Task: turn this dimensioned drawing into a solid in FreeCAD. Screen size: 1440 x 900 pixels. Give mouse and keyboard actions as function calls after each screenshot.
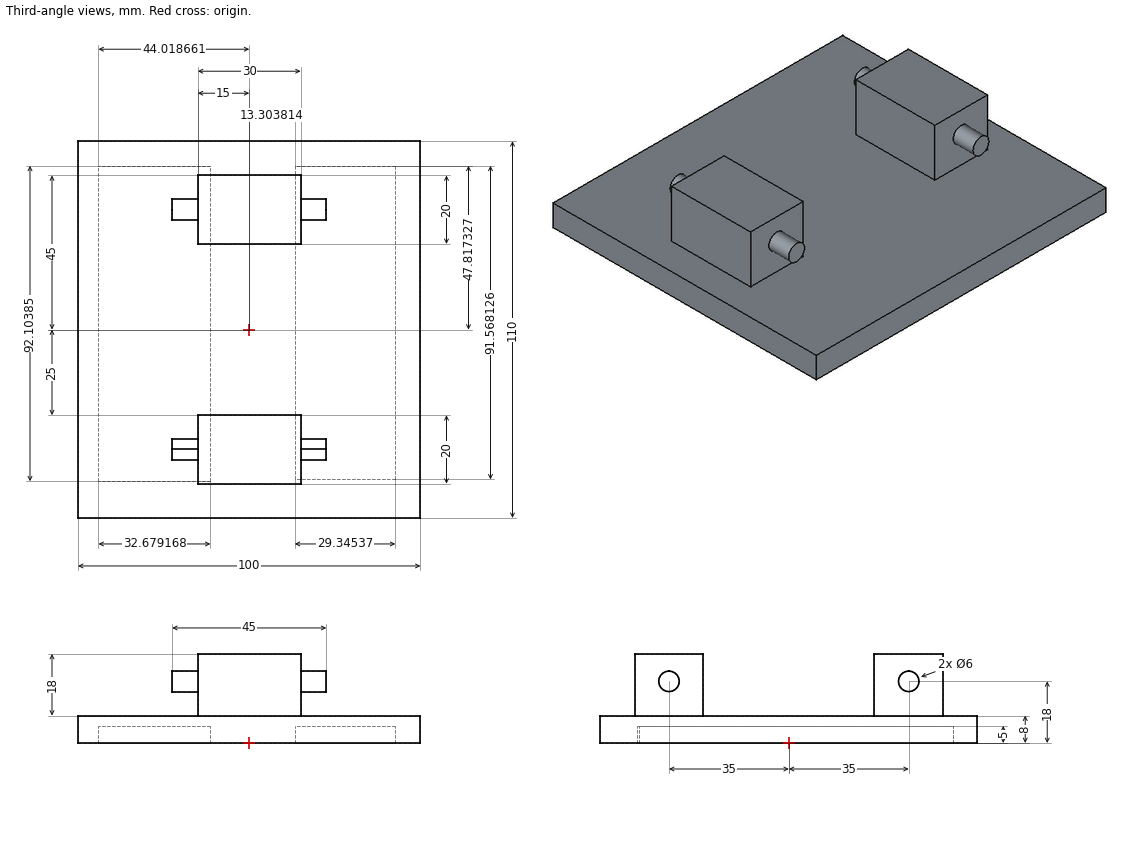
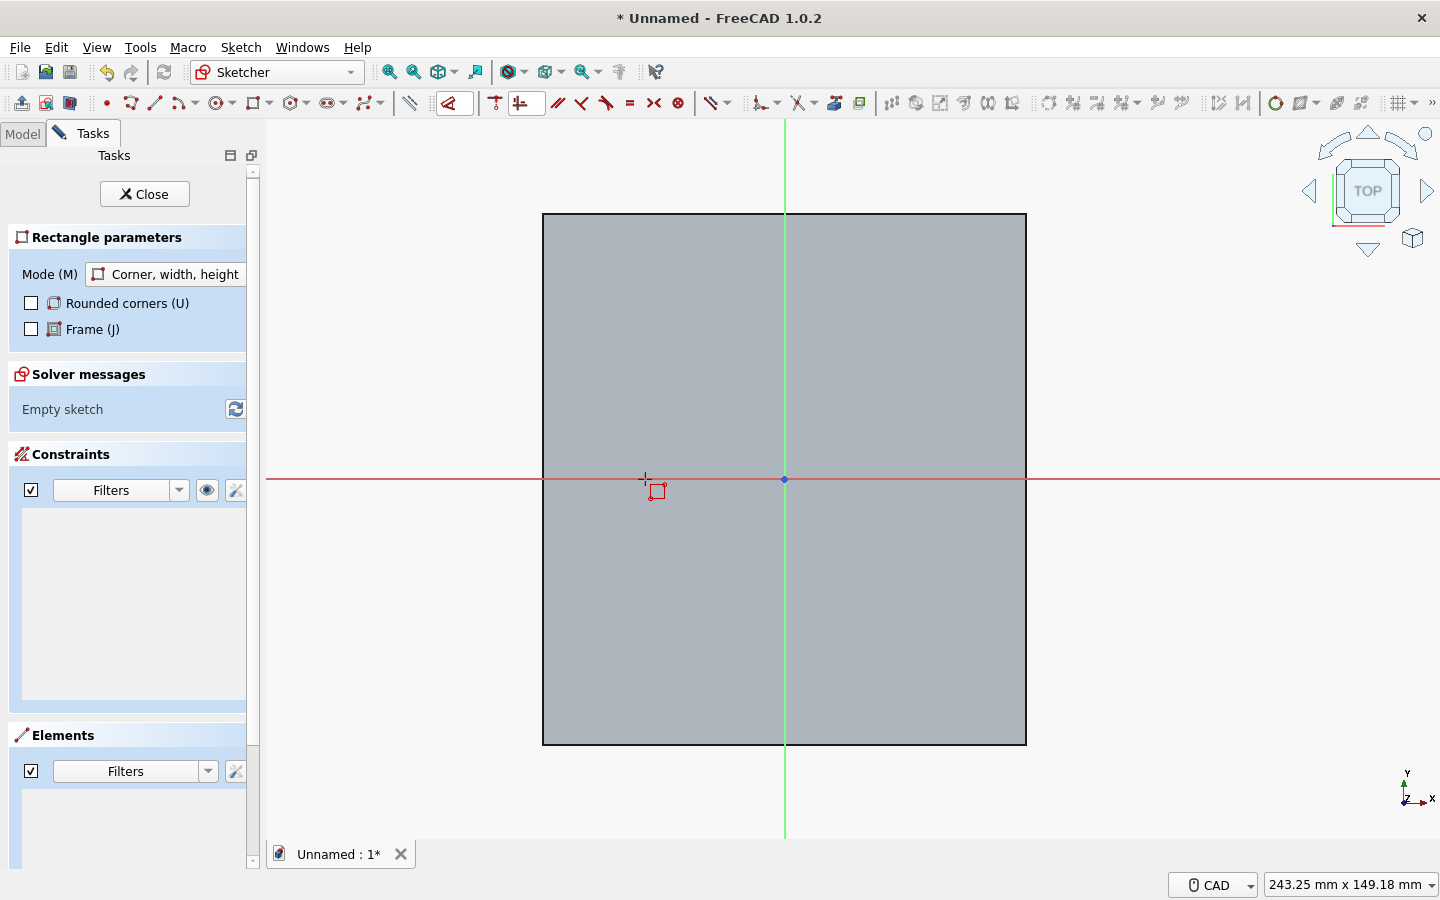
click(712, 262)
move(857, 359)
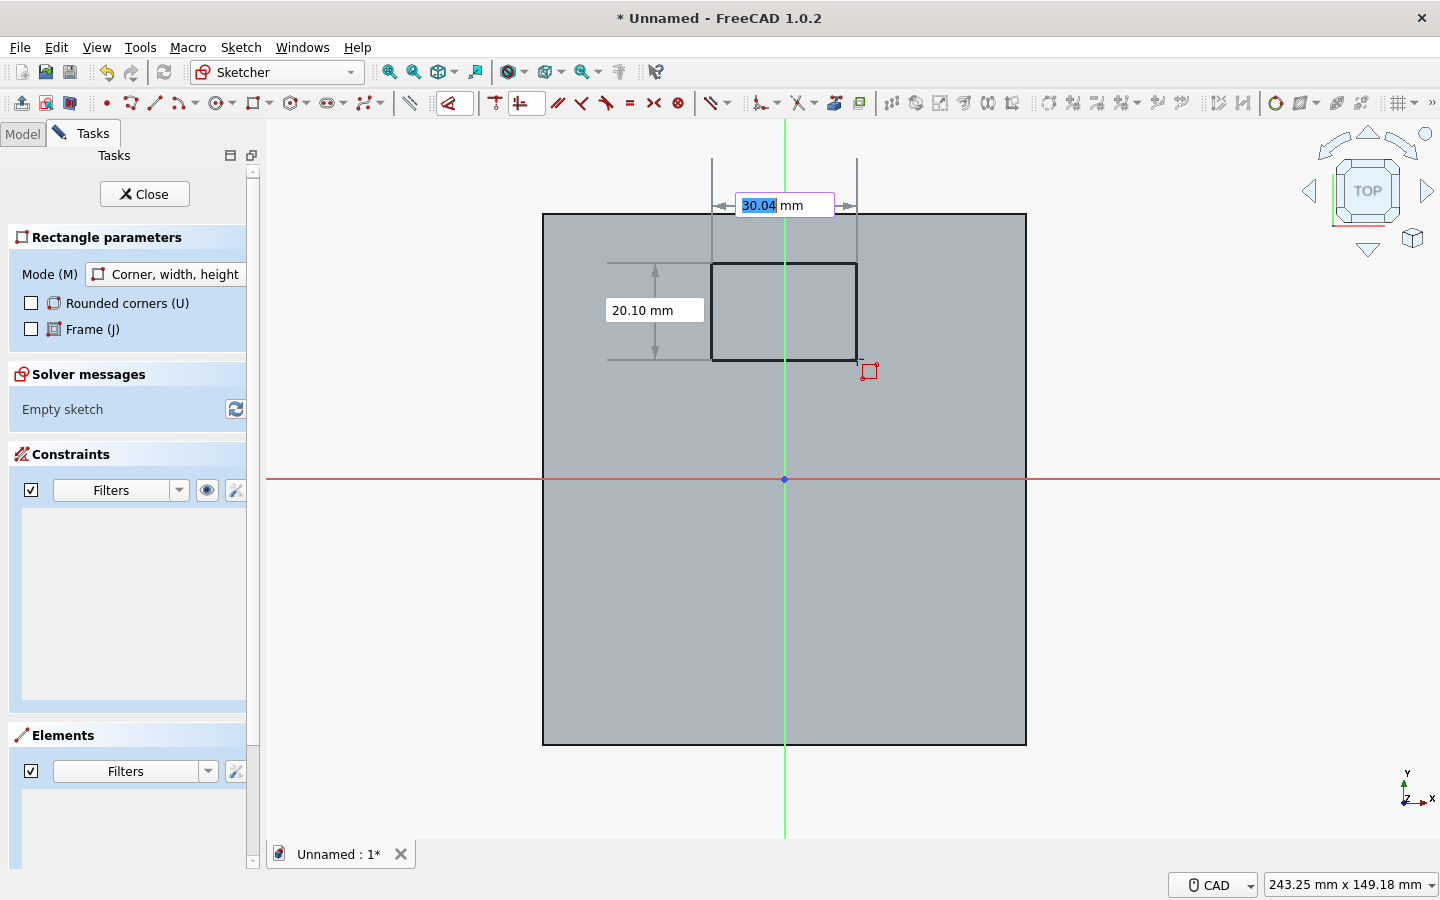
text(30)
key(Tab)
text(20)
key(Return)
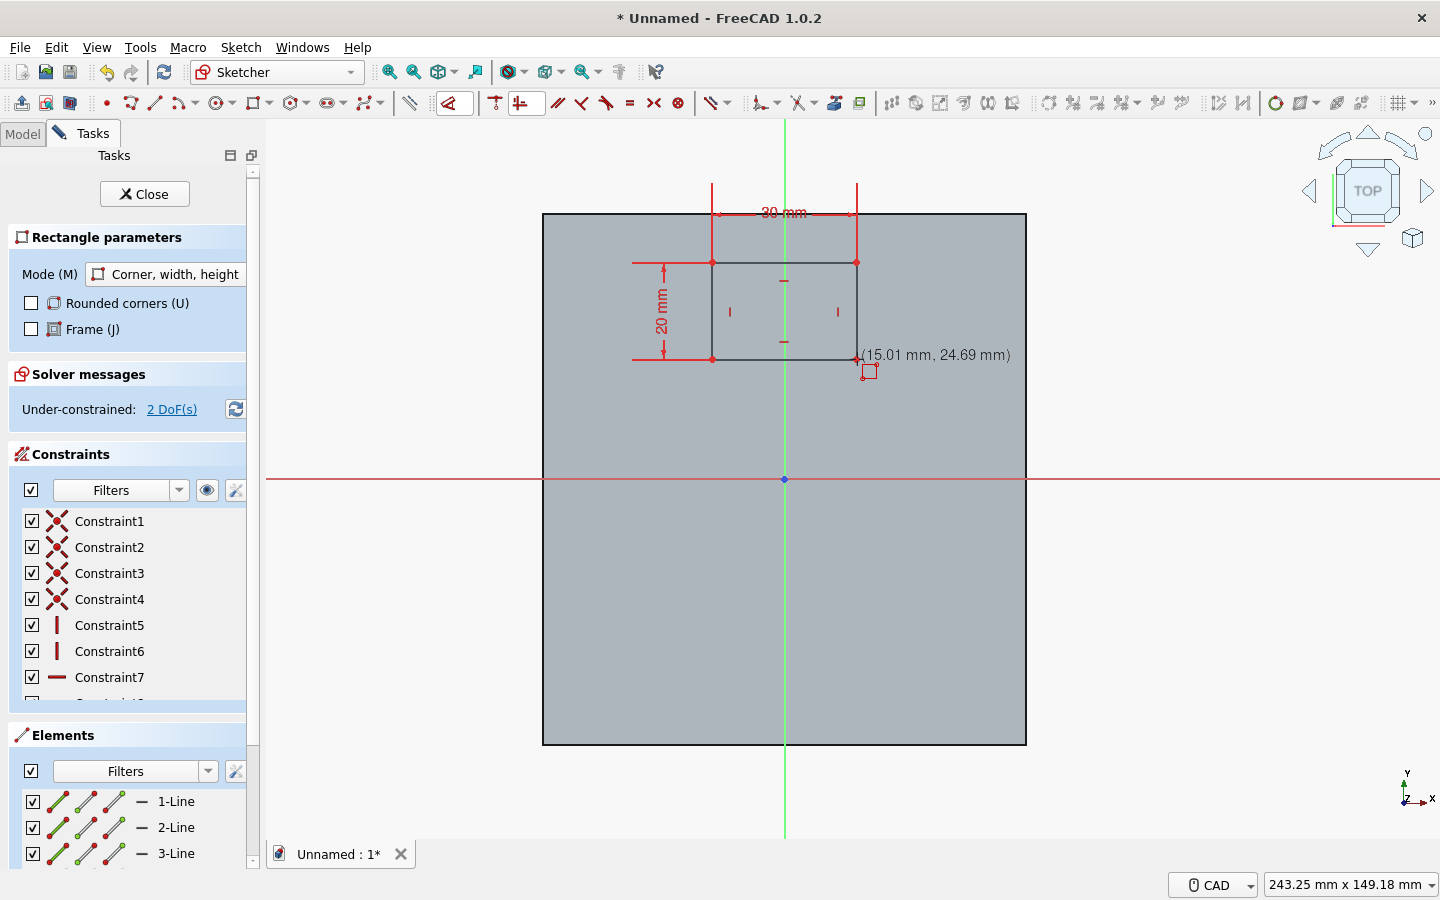
click(712, 600)
move(857, 696)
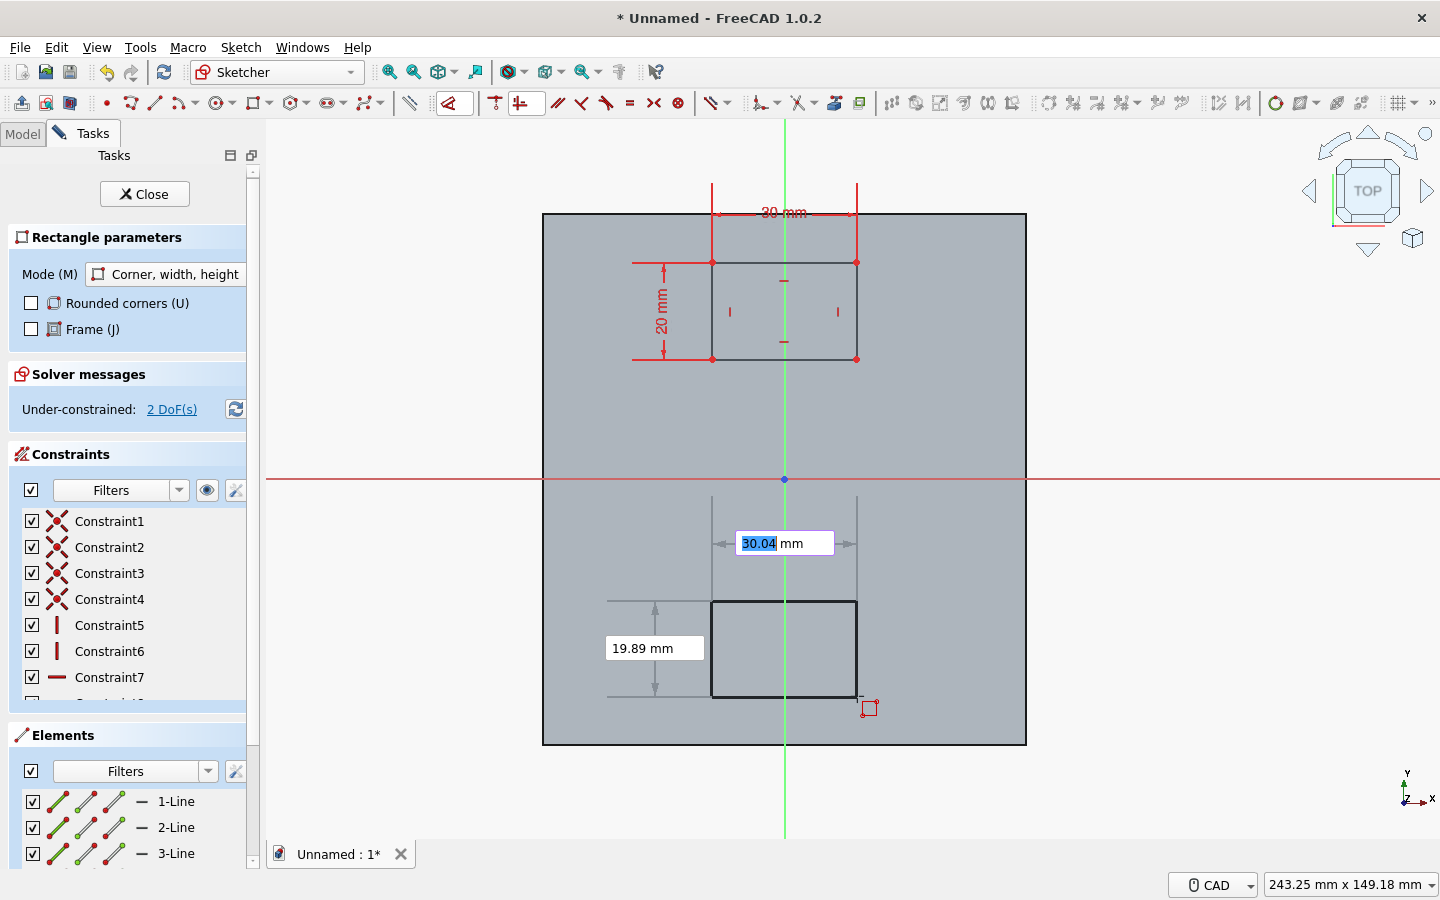
text(30)
key(Tab)
text(20)
key(Return)
key(Escape)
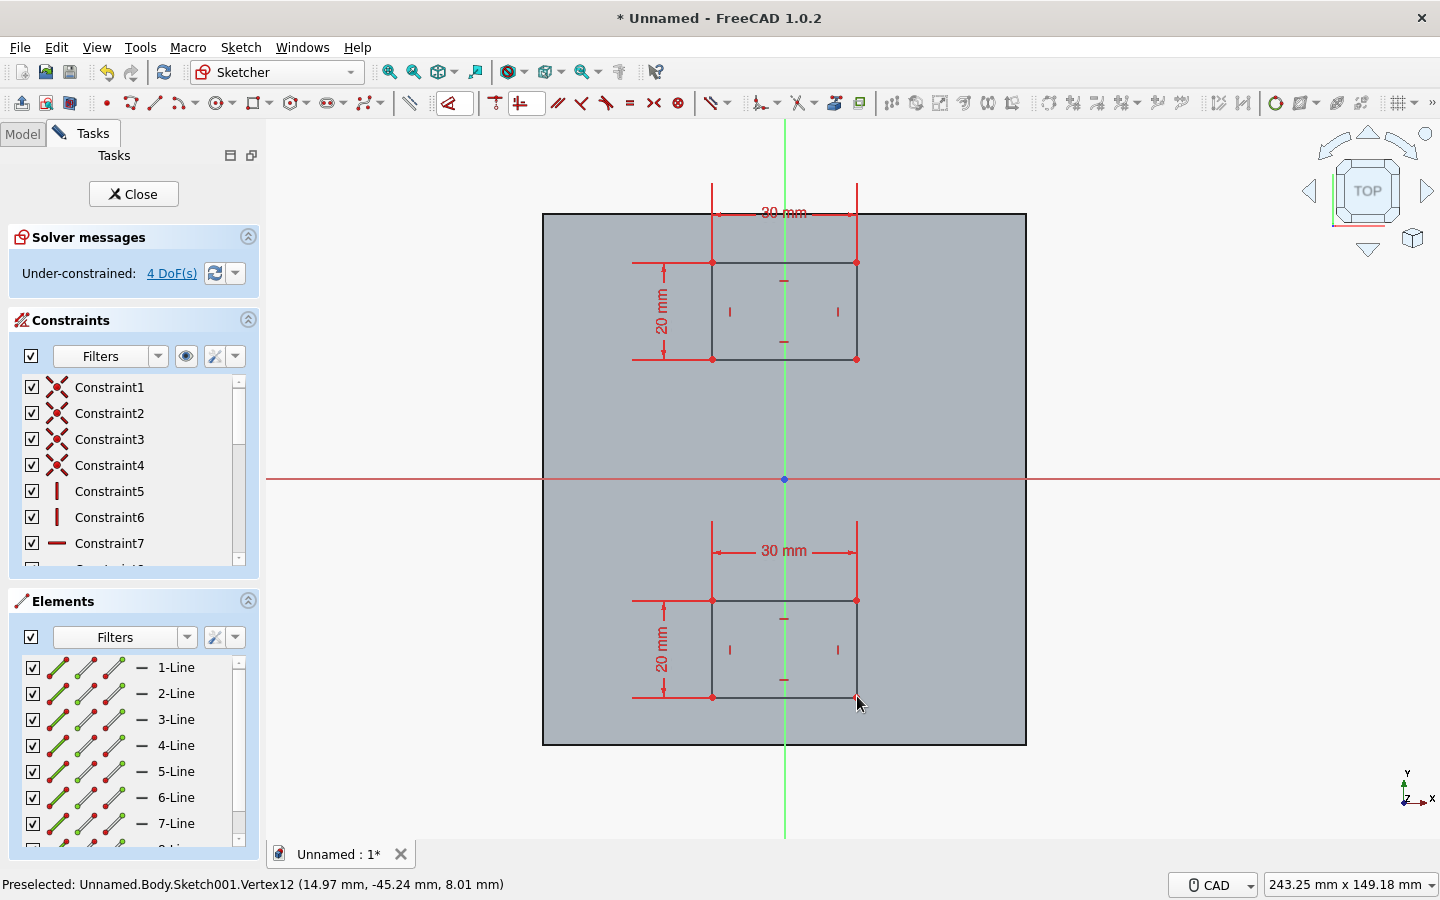
key(d)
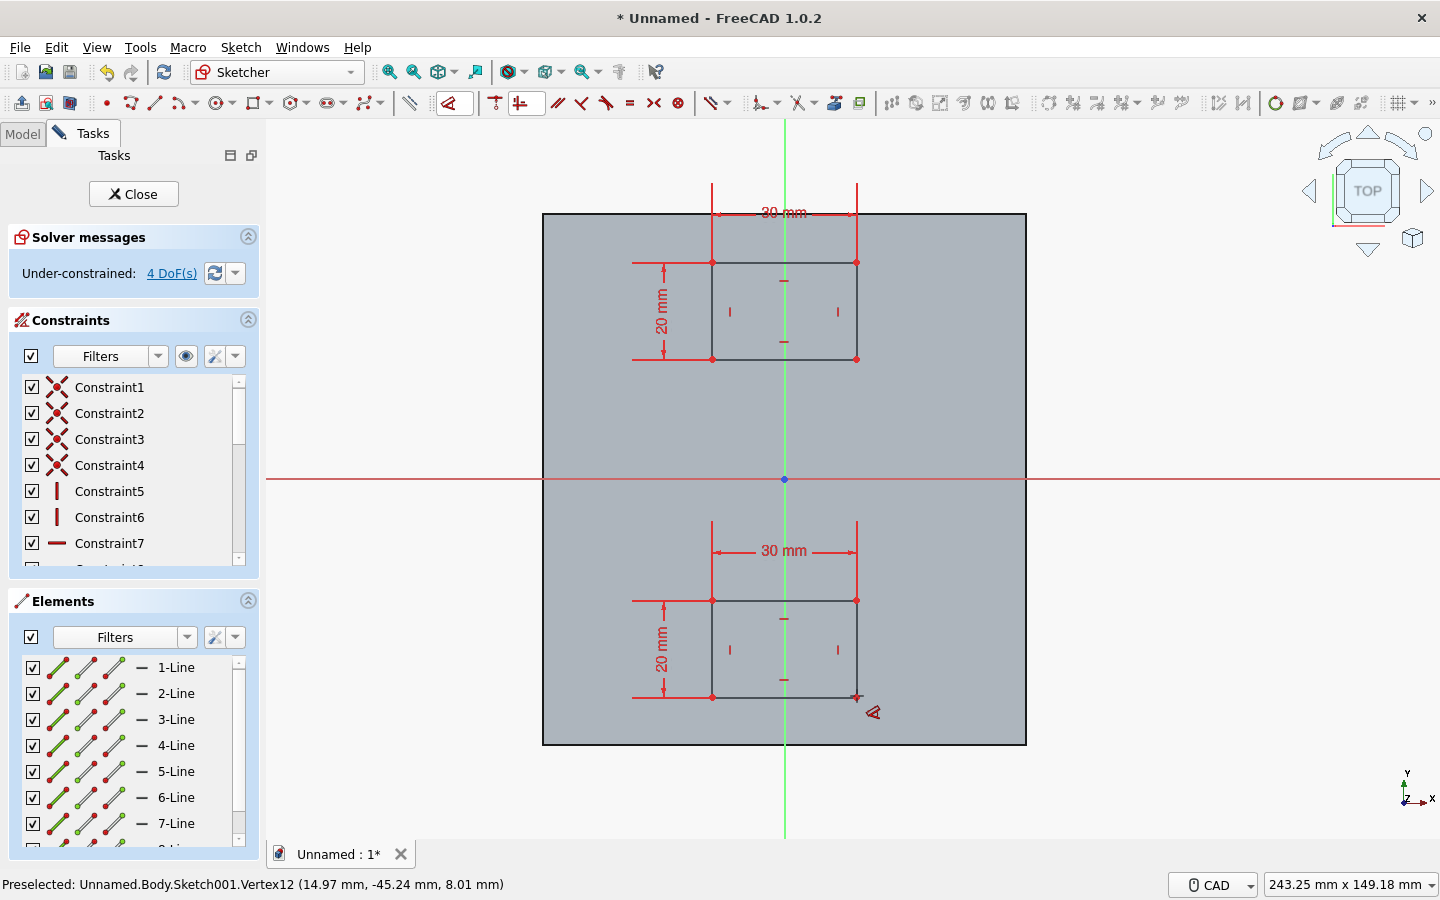
click(712, 263)
click(748, 229)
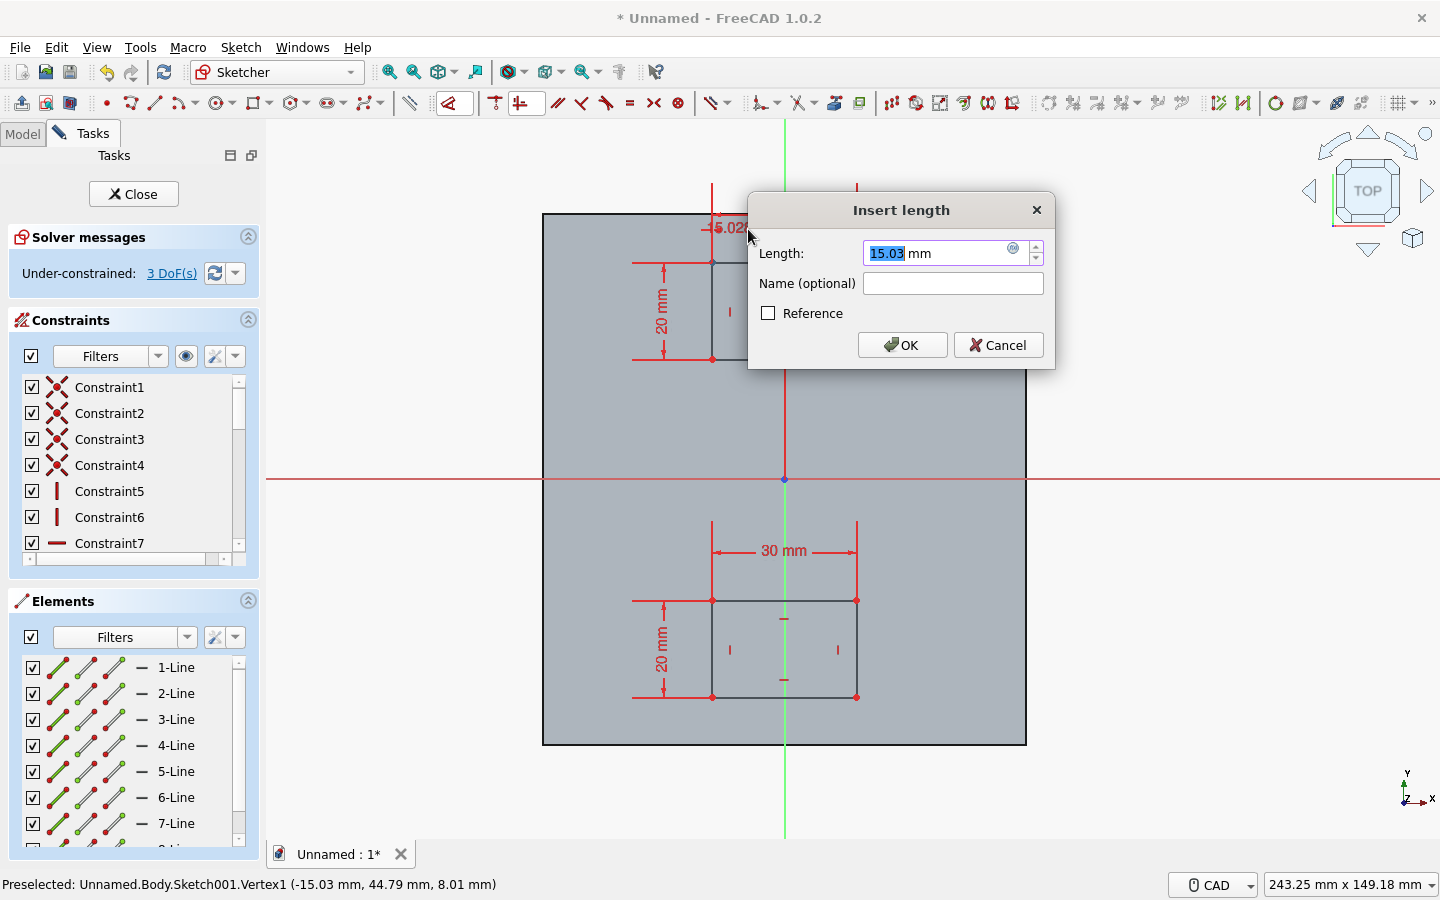
text(15)
key(Return)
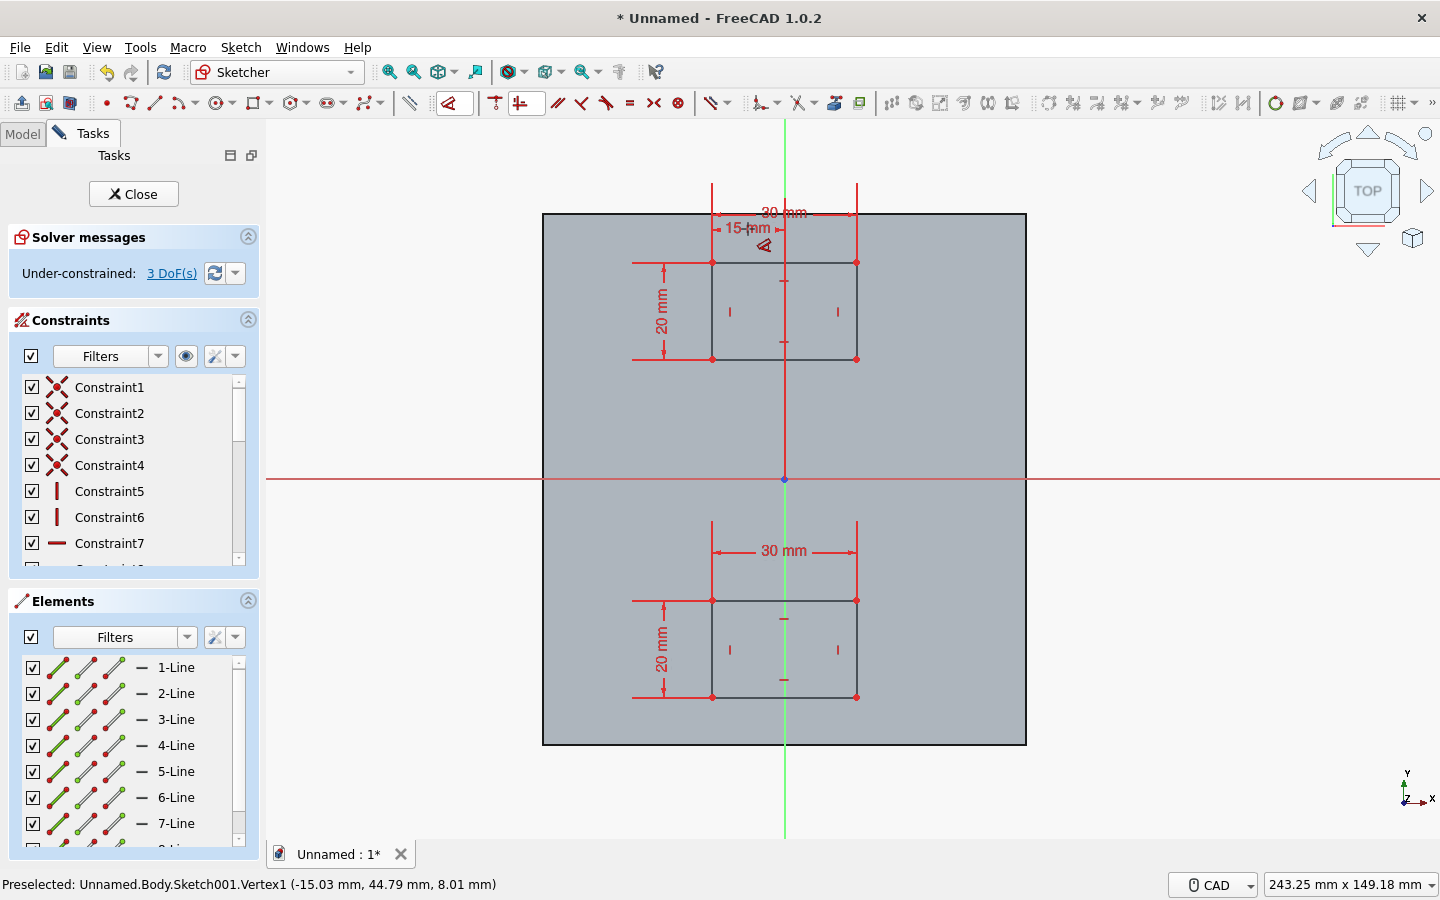
click(712, 263)
click(678, 371)